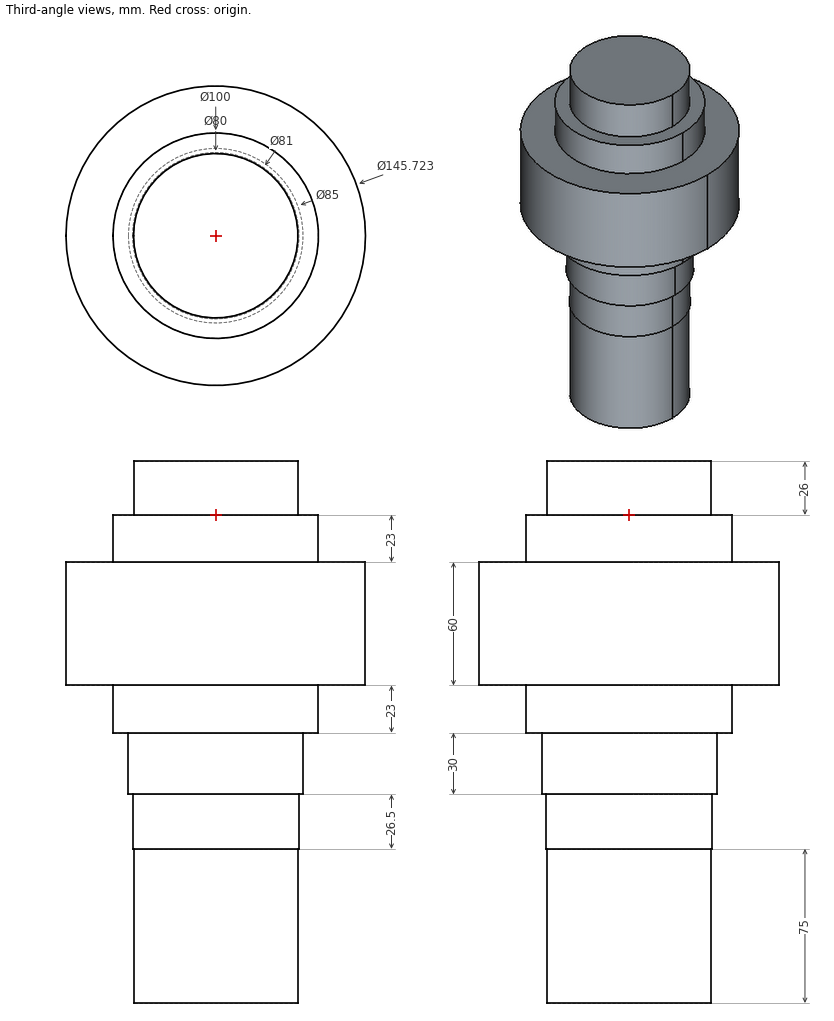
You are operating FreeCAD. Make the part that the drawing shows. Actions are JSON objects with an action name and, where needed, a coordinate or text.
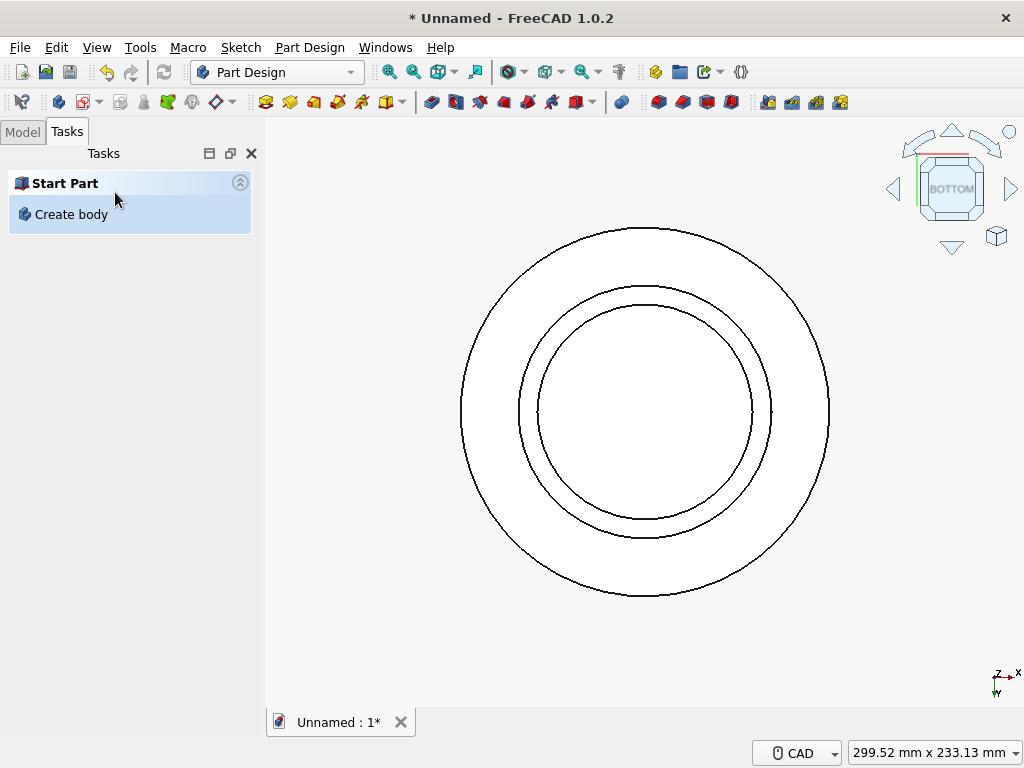
{"action": "left_click", "coordinate": [645, 411]}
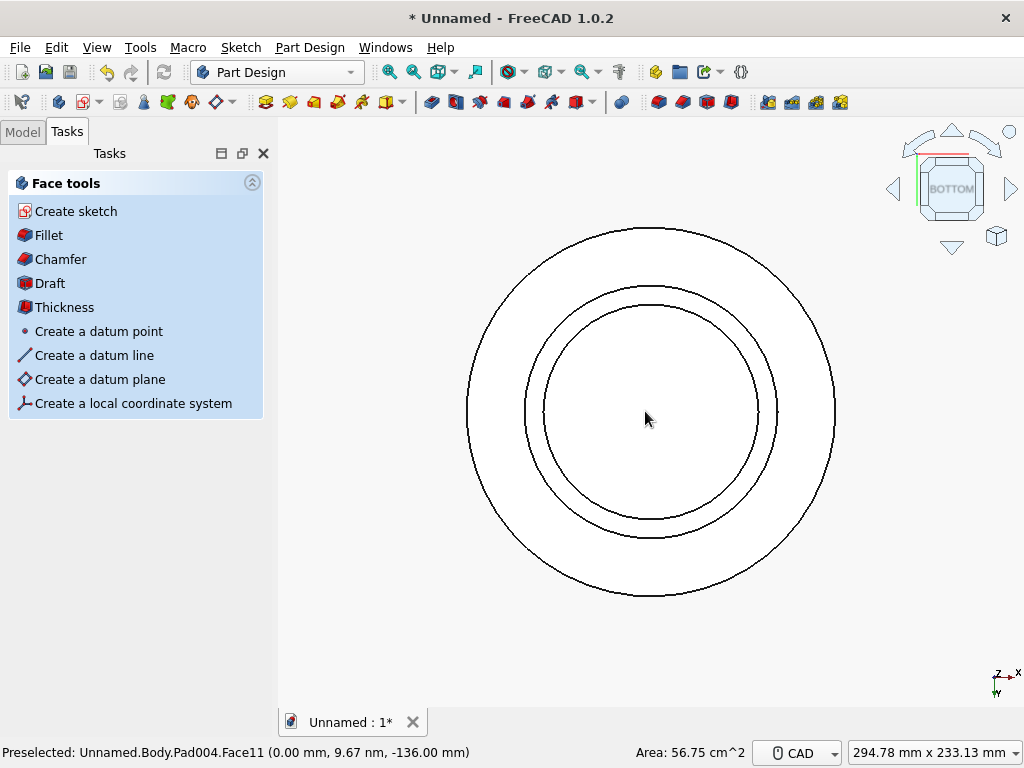
{"action": "left_click", "coordinate": [84, 102]}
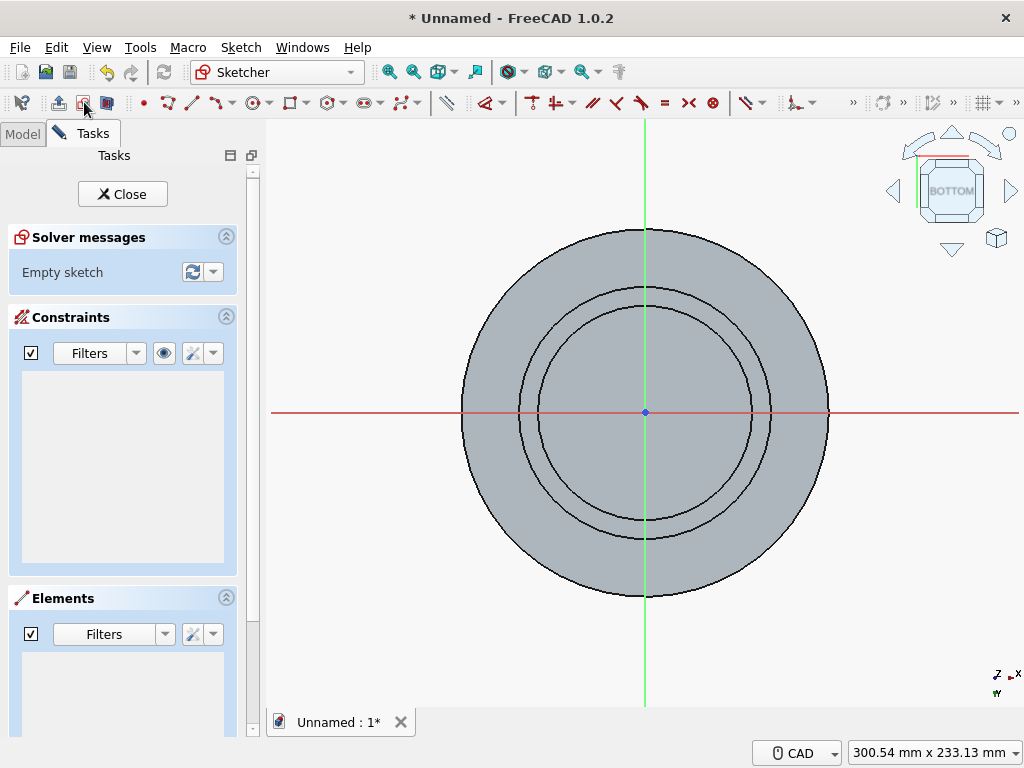
{"action": "scroll", "coordinate": [728, 413], "scroll_direction": "up", "scroll_amount": 3}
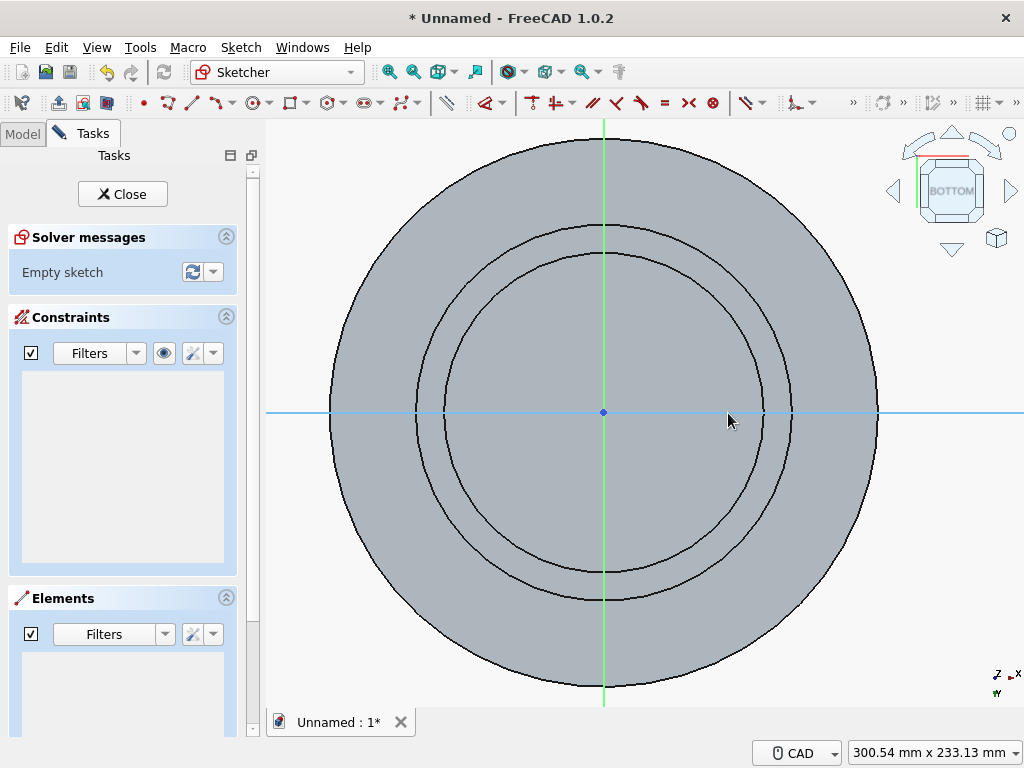
{"action": "left_click", "coordinate": [254, 104]}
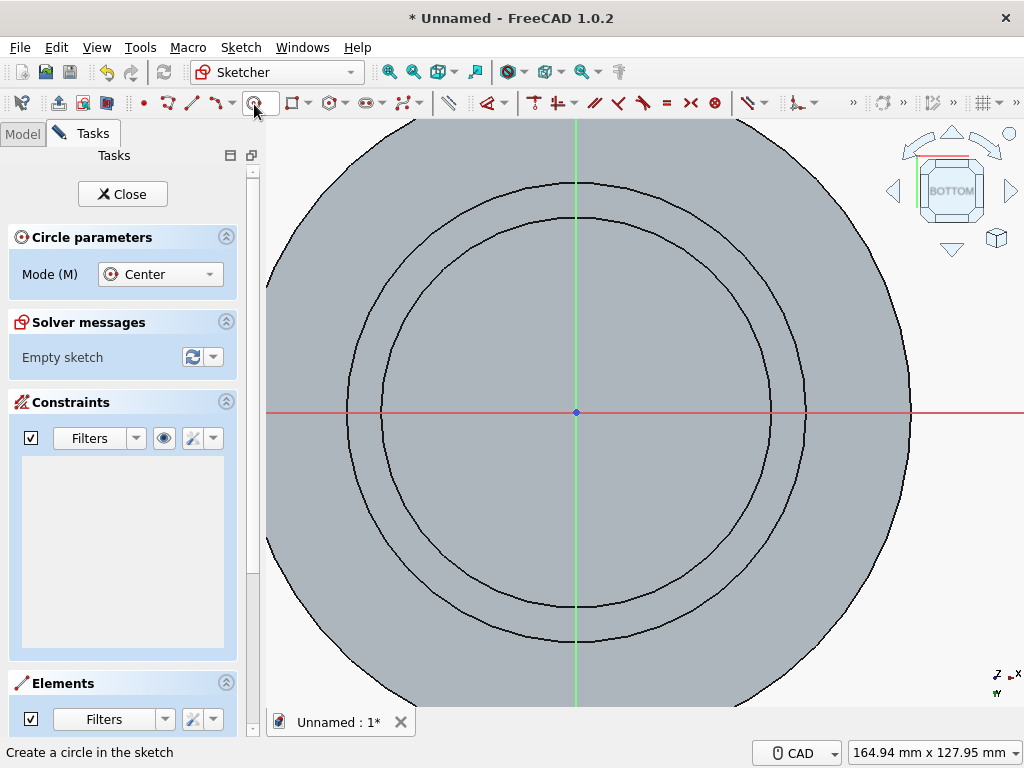
{"action": "left_click", "coordinate": [576, 413]}
{"action": "left_click", "coordinate": [708, 281]}
{"action": "key", "text": "Escape"}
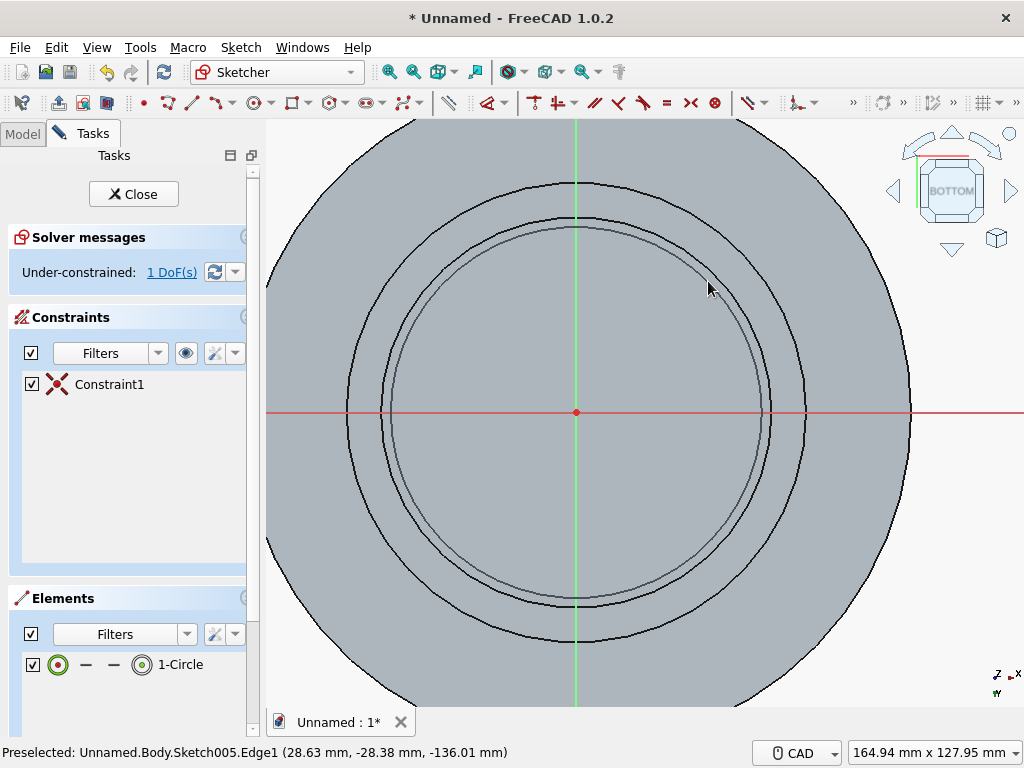
{"action": "left_click", "coordinate": [488, 104]}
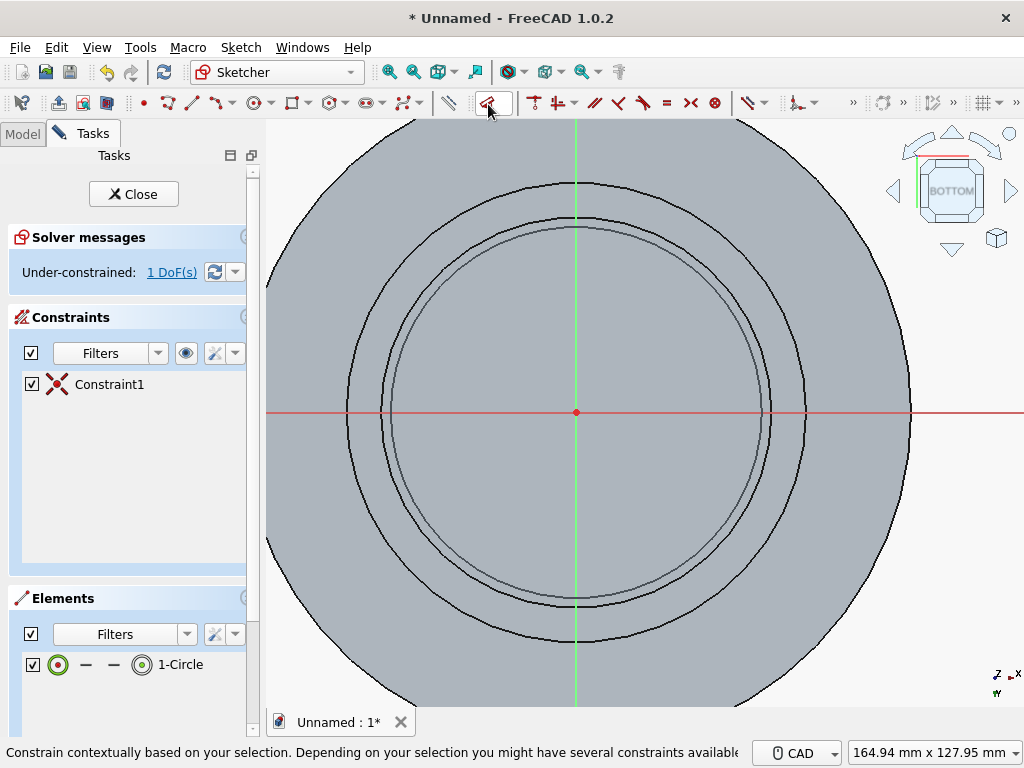
{"action": "left_click", "coordinate": [707, 281]}
{"action": "left_click", "coordinate": [730, 258]}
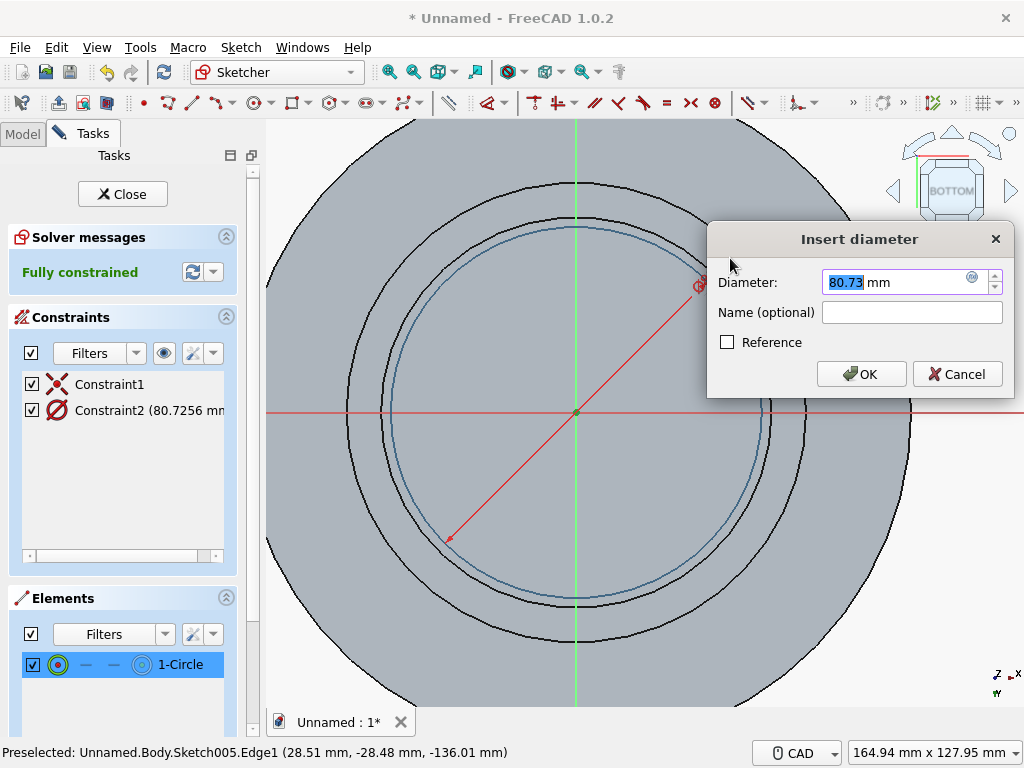
{"action": "type", "text": "81"}
{"action": "key", "text": "Return"}
{"action": "key", "text": "Escape"}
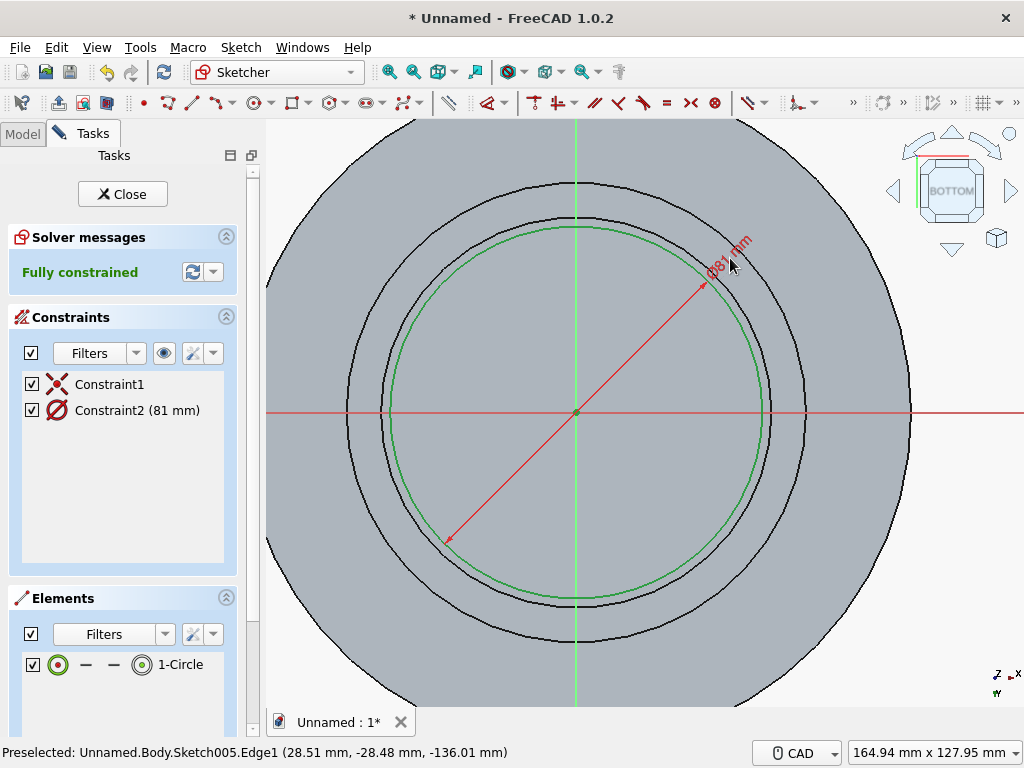
{"action": "left_click", "coordinate": [123, 194]}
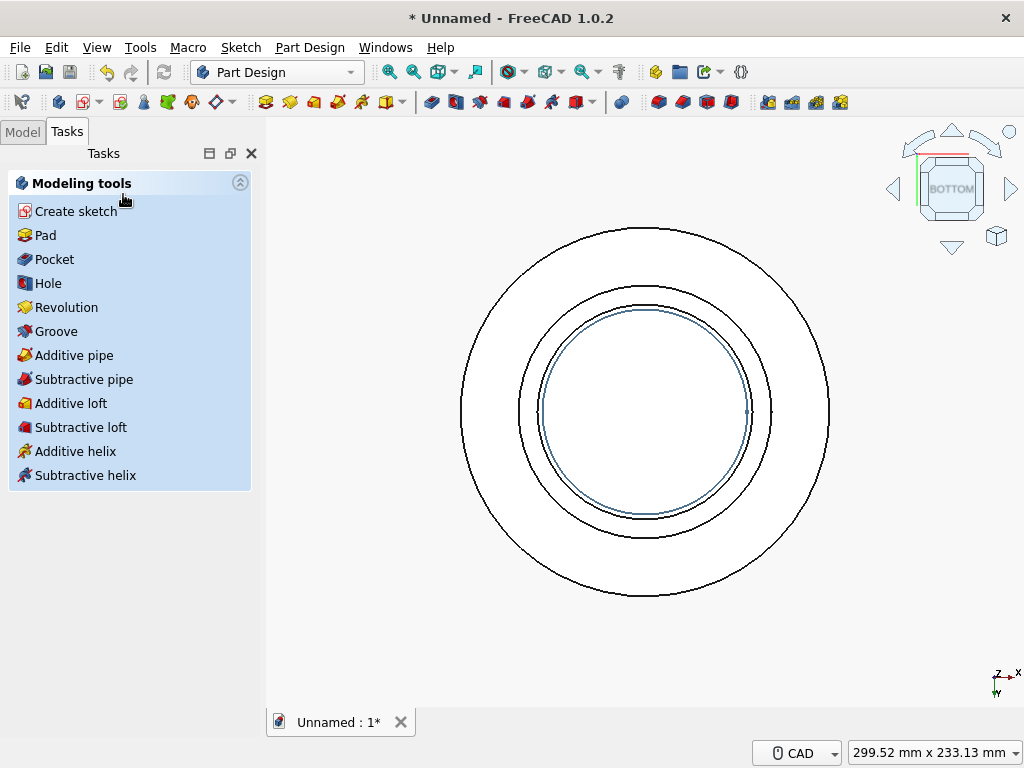
{"action": "left_click", "coordinate": [266, 102]}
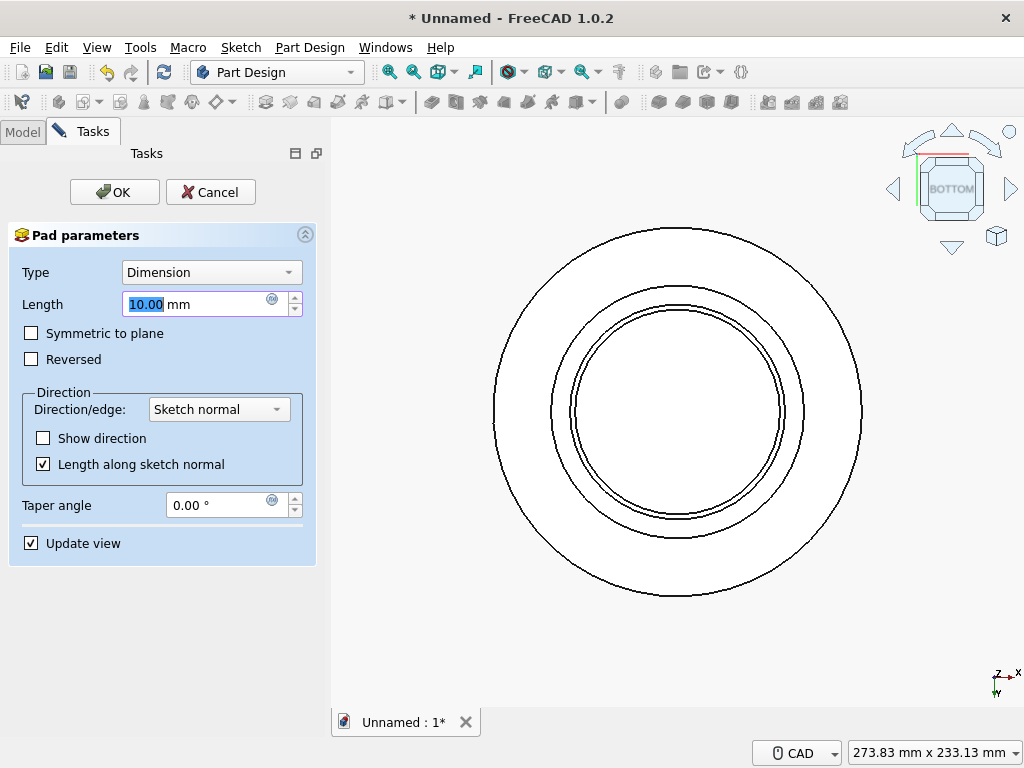
{"action": "type", "text": "26.5"}
{"action": "key", "text": "Tab"}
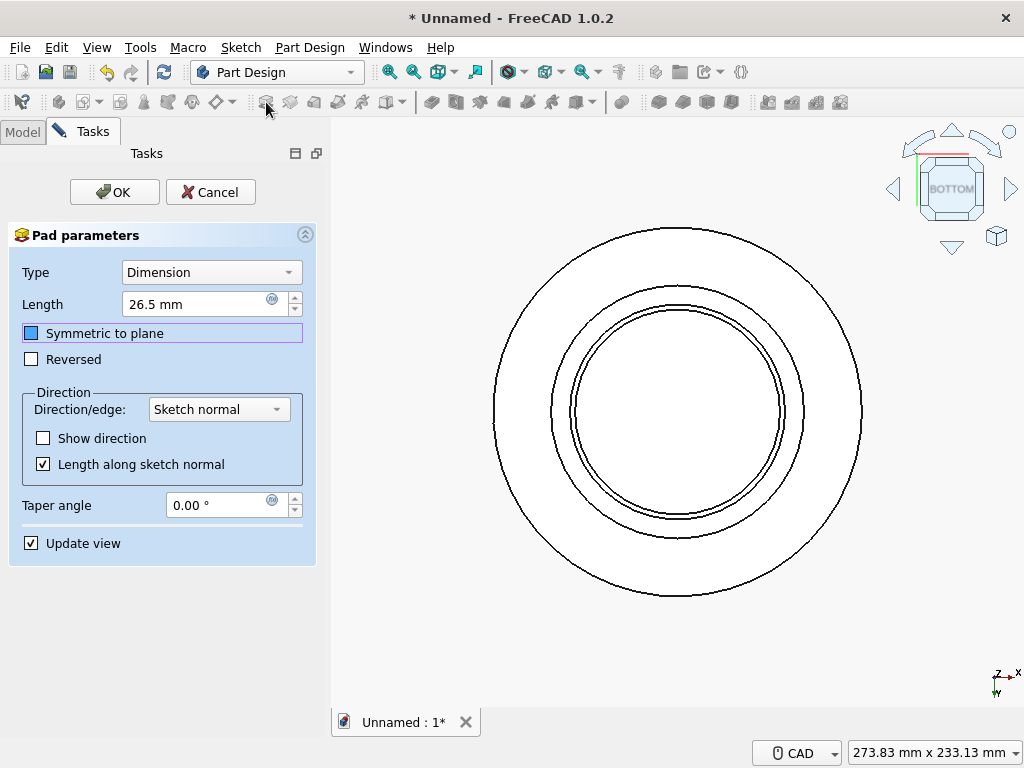
{"action": "left_click", "coordinate": [115, 192]}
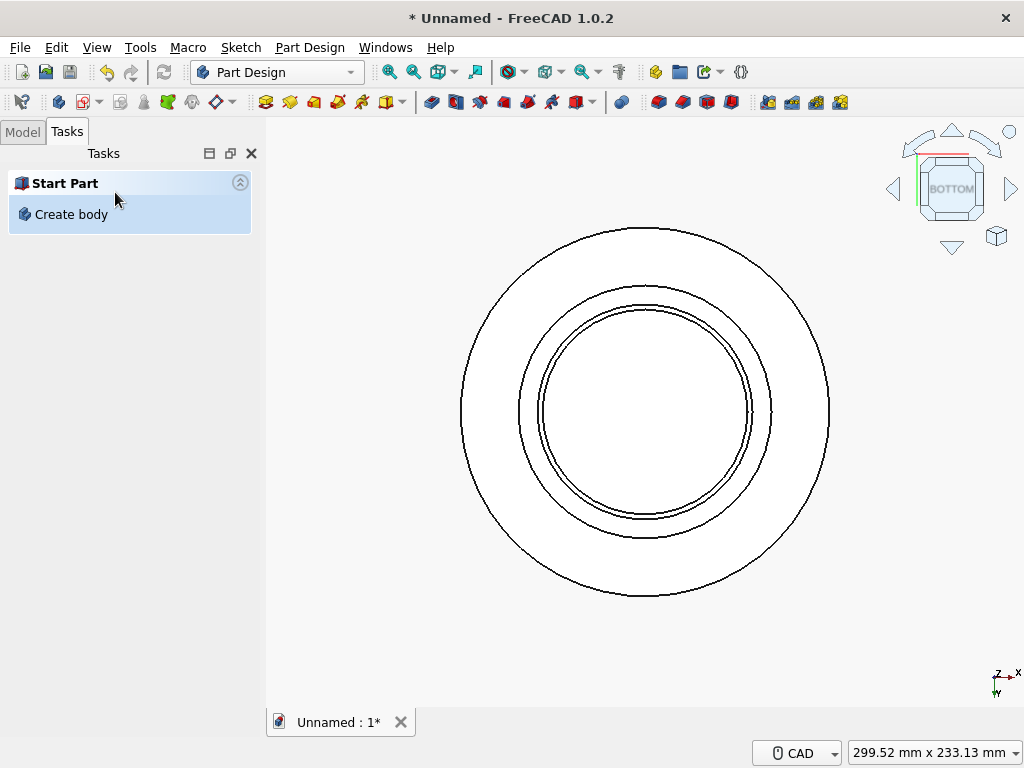
{"action": "left_click", "coordinate": [23, 131]}